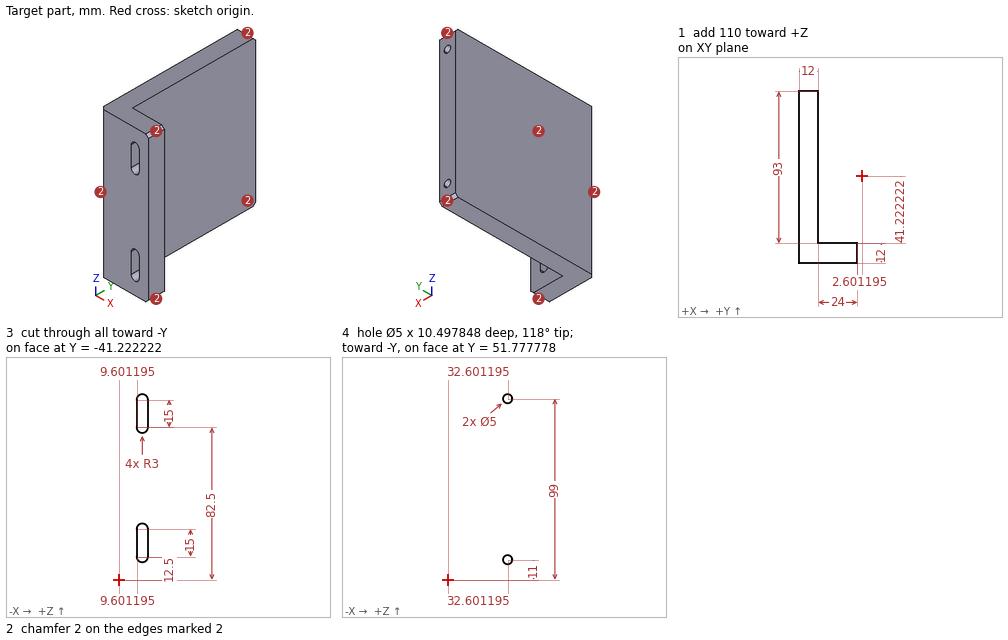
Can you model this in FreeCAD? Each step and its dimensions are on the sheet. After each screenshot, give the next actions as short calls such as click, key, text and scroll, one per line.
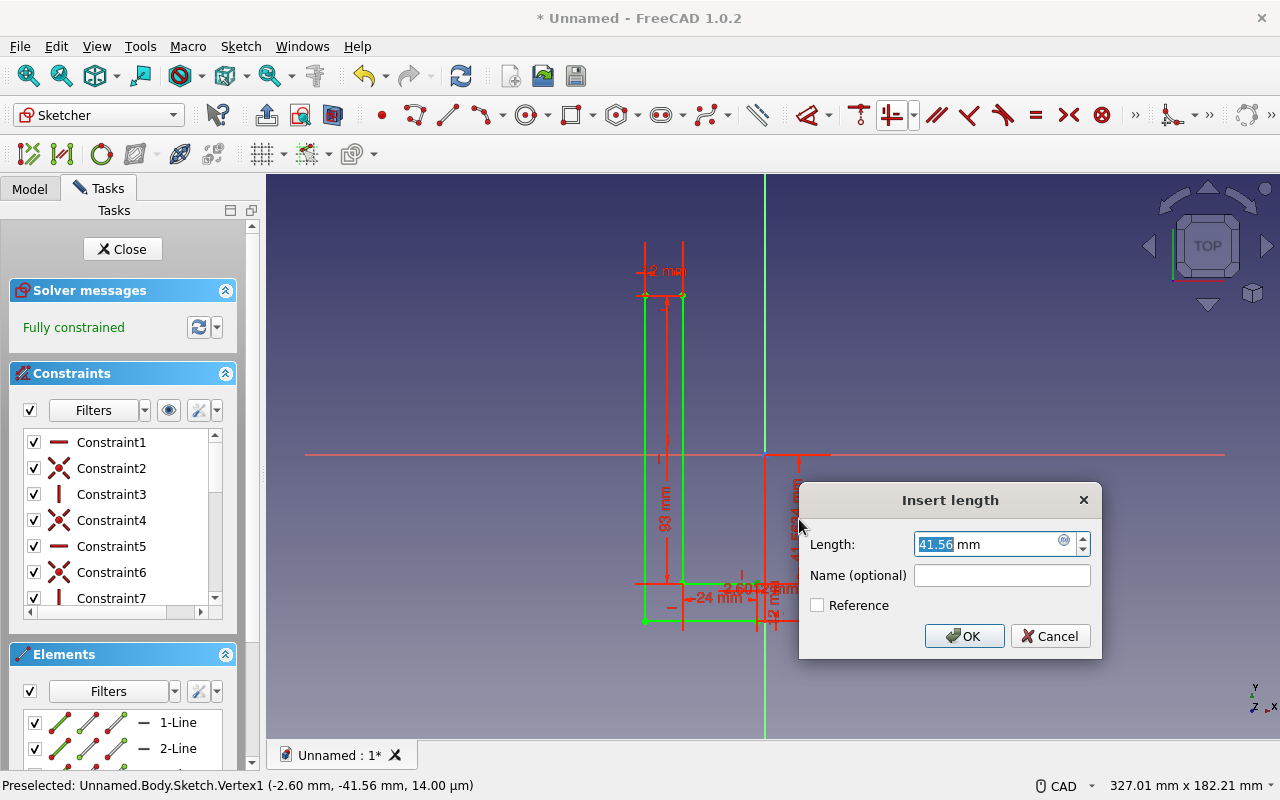
text(41.222222)
key(Return)
key(Escape)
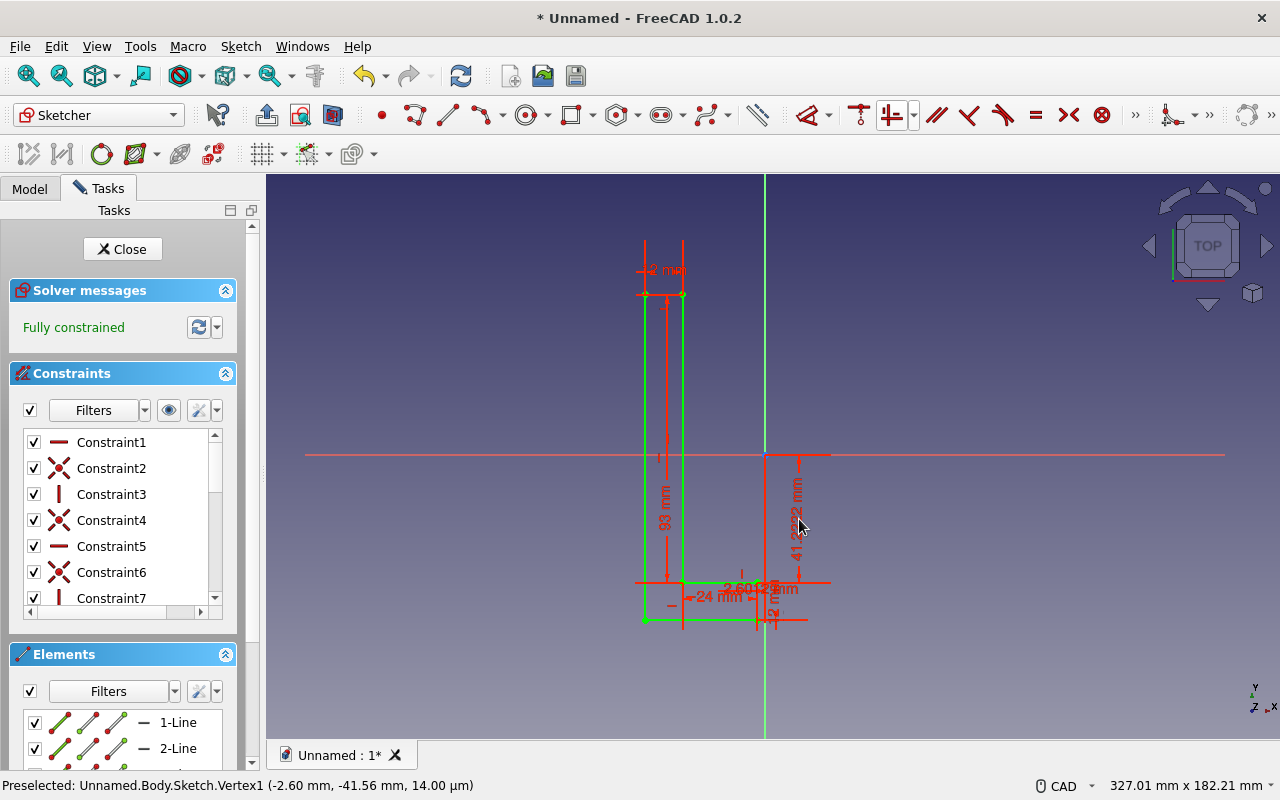
click(123, 249)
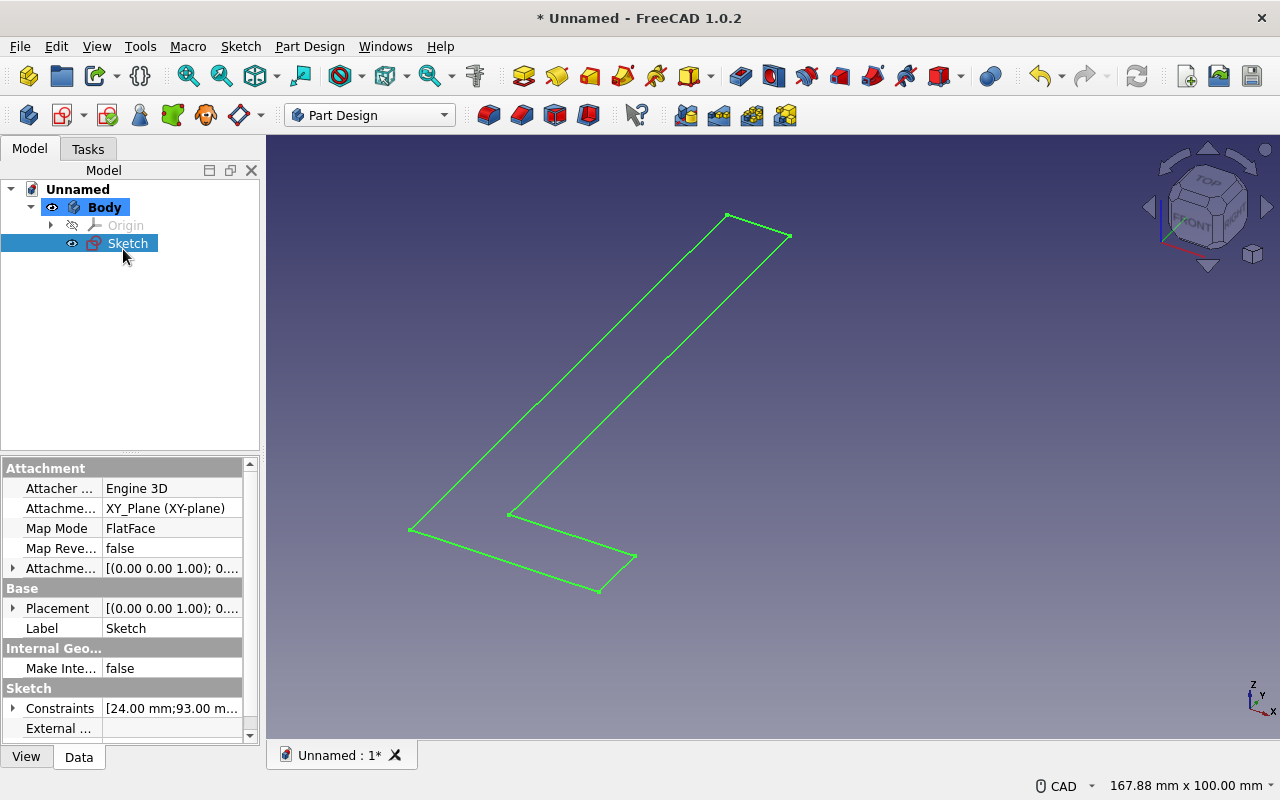
click(524, 76)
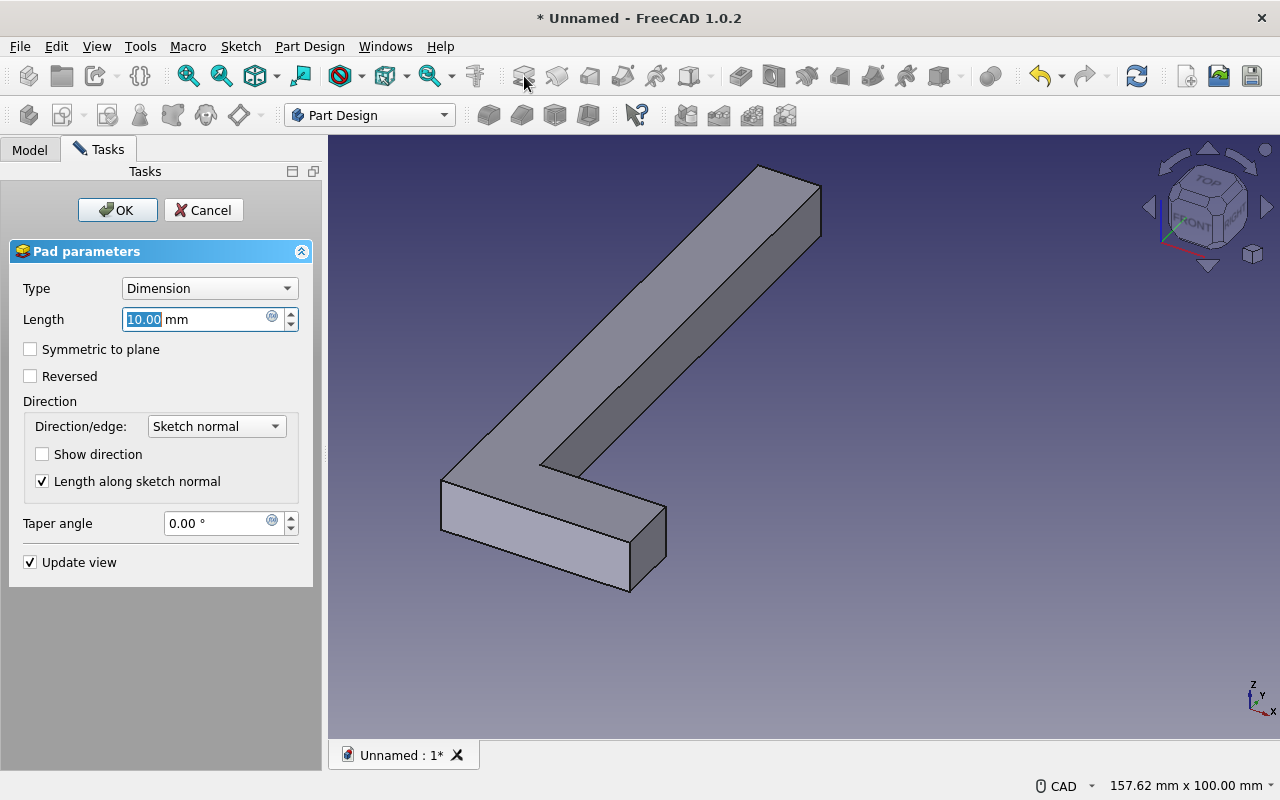
text(110)
key(Tab)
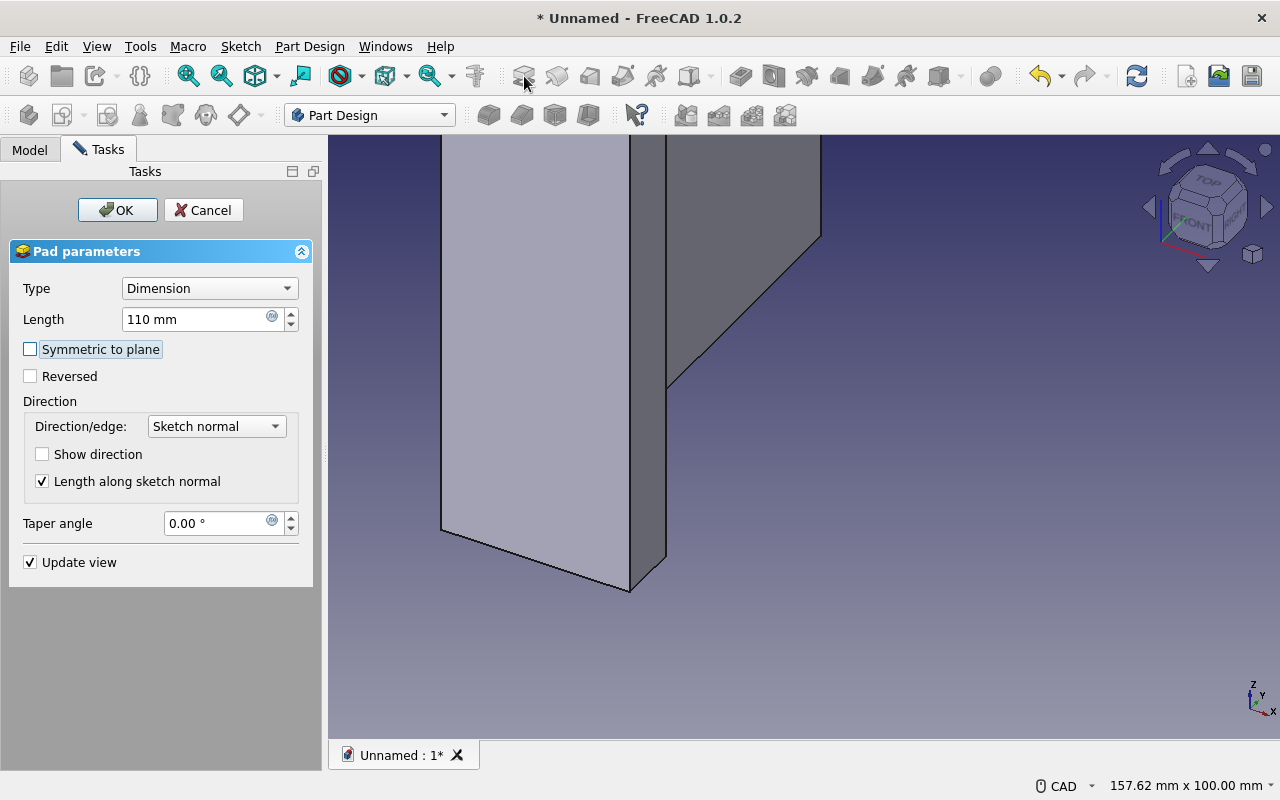
click(118, 210)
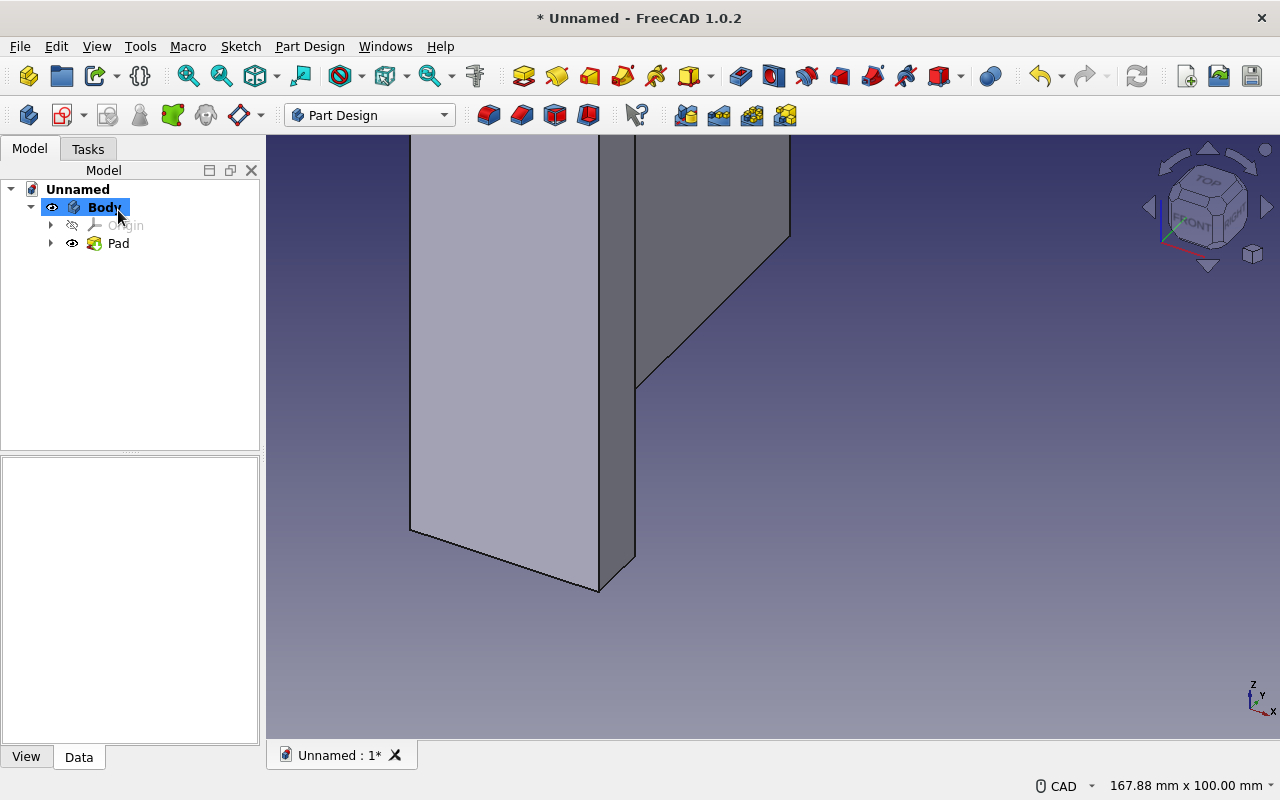
click(189, 76)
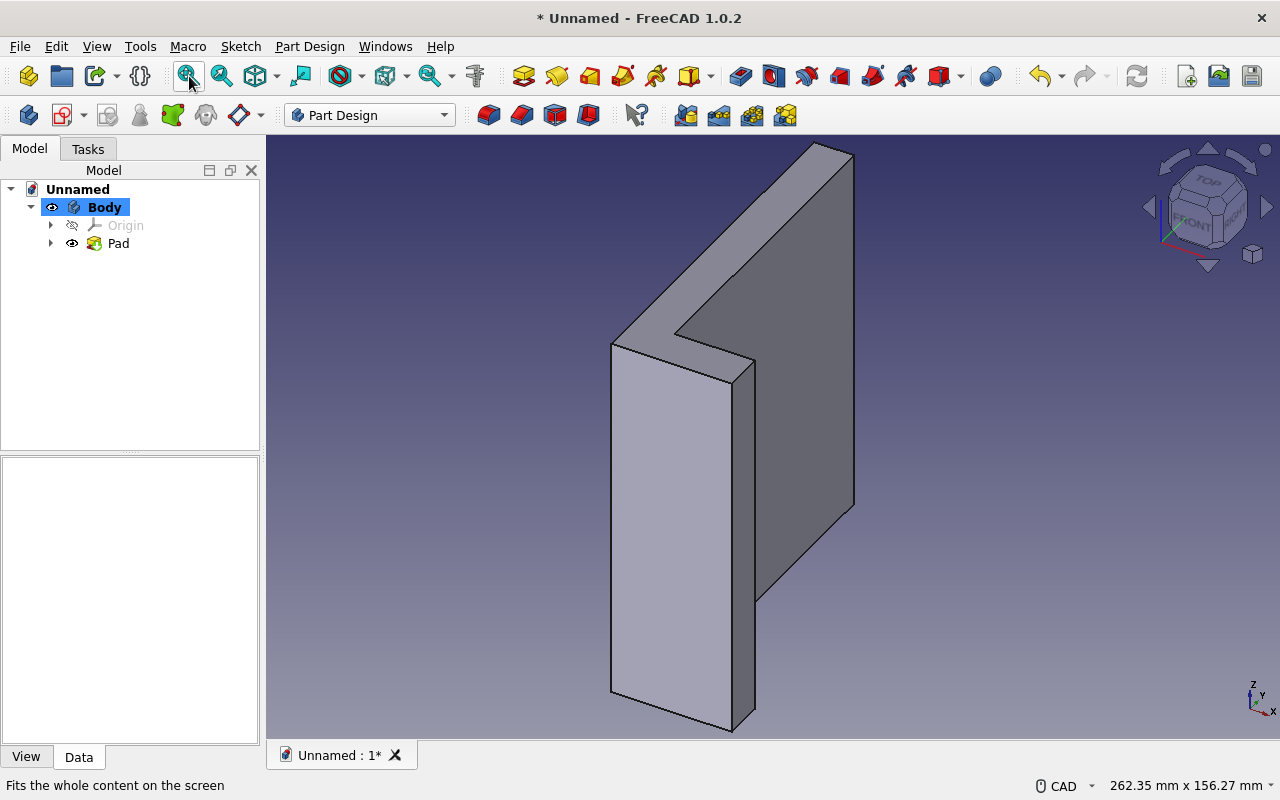
click(743, 371)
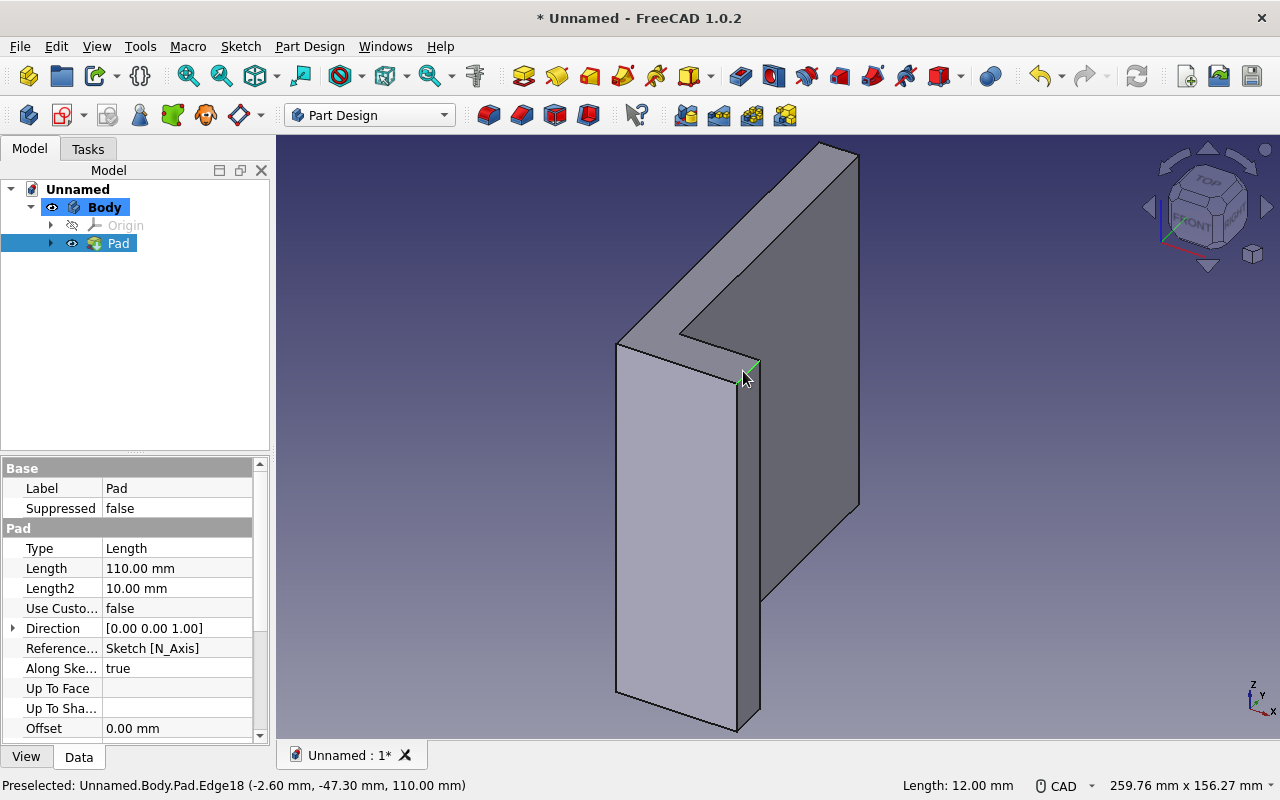
key(0)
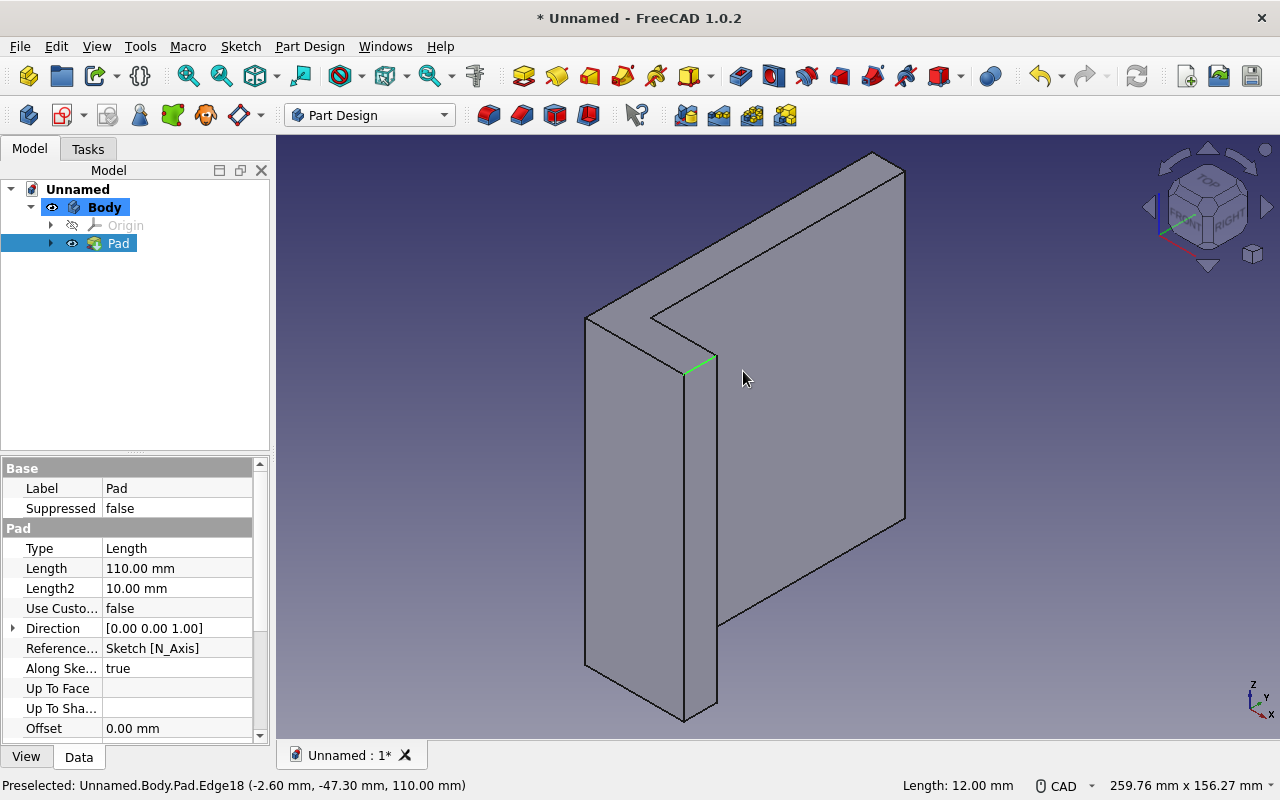
key(2)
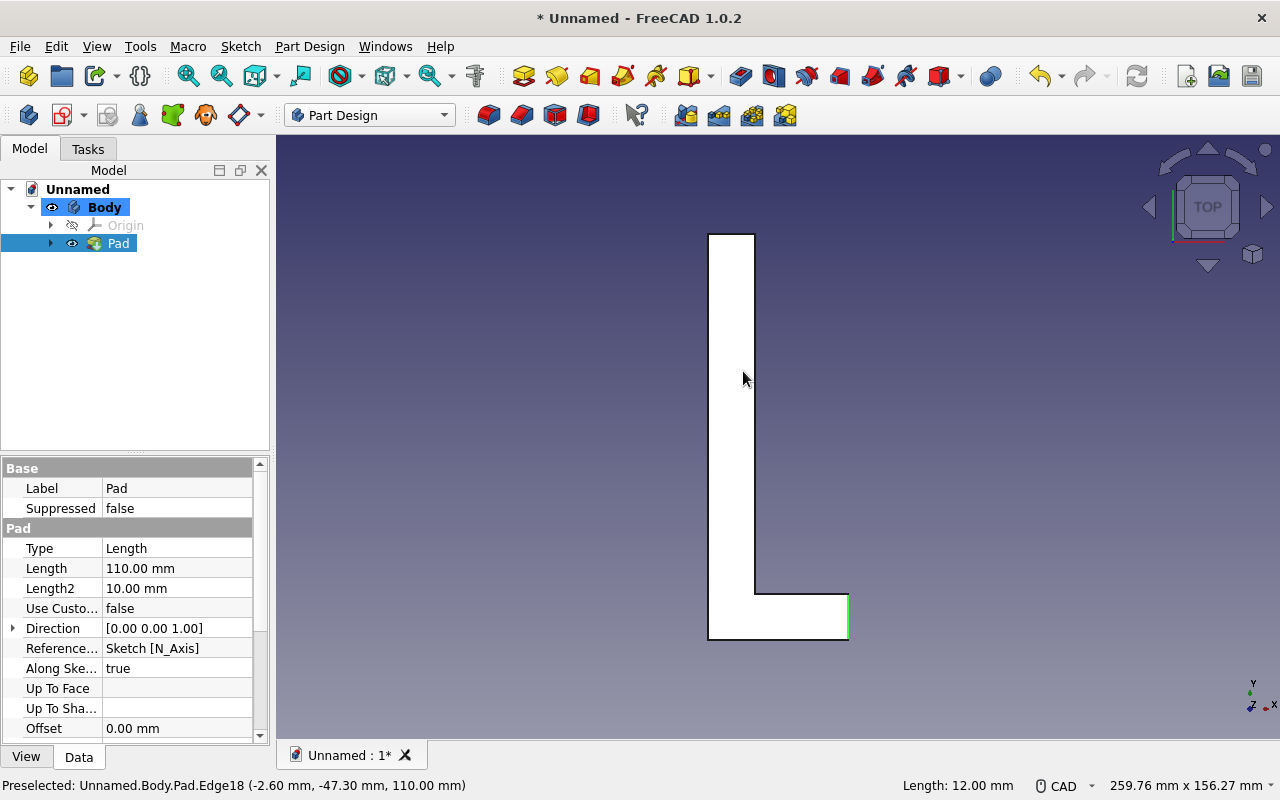
click(732, 233, ctrl)